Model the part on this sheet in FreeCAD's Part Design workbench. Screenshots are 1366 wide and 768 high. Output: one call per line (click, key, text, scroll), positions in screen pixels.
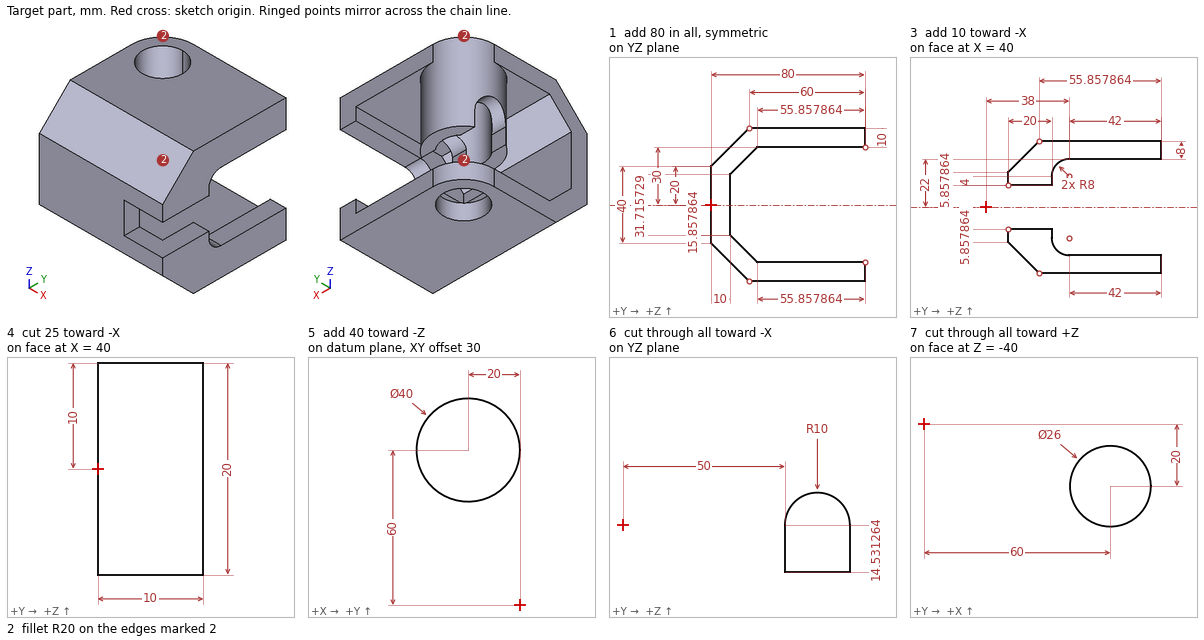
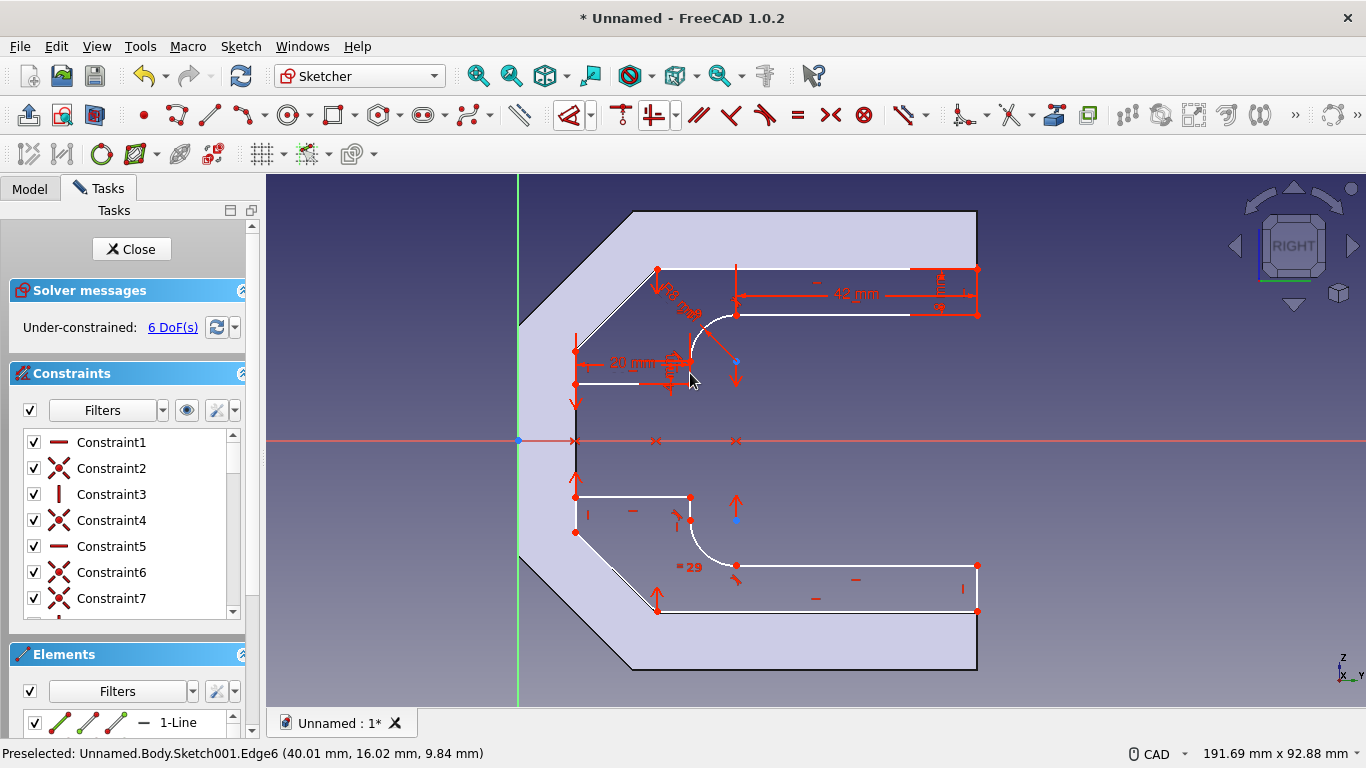
click(905, 566)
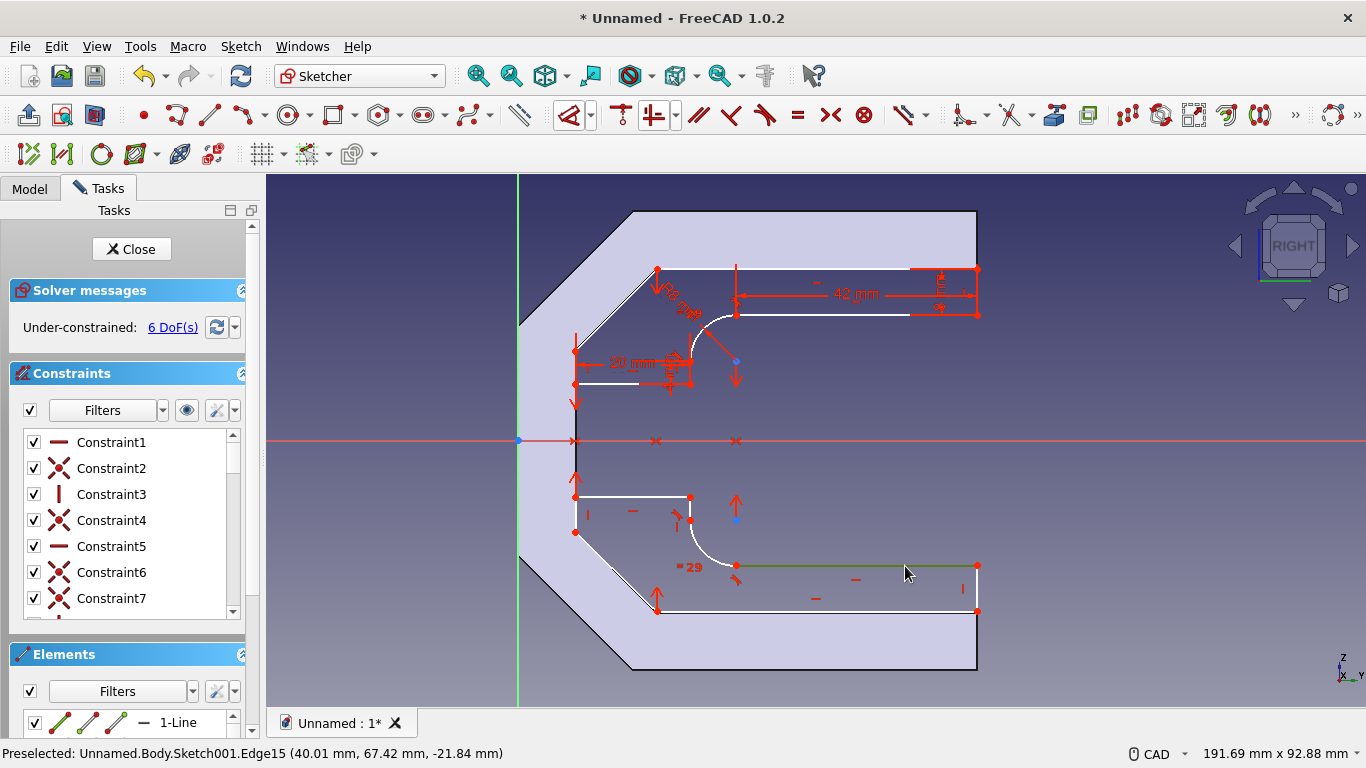
key(l)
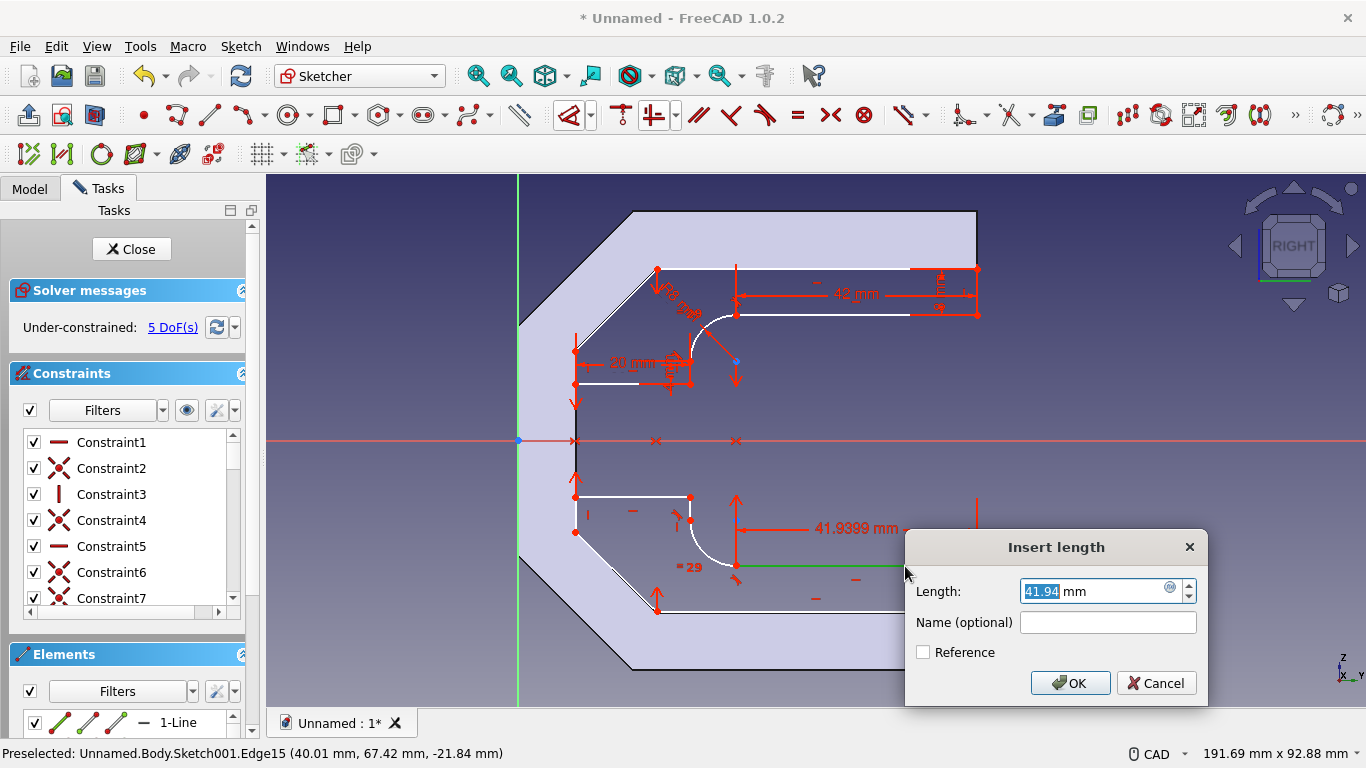
text(42)
key(Return)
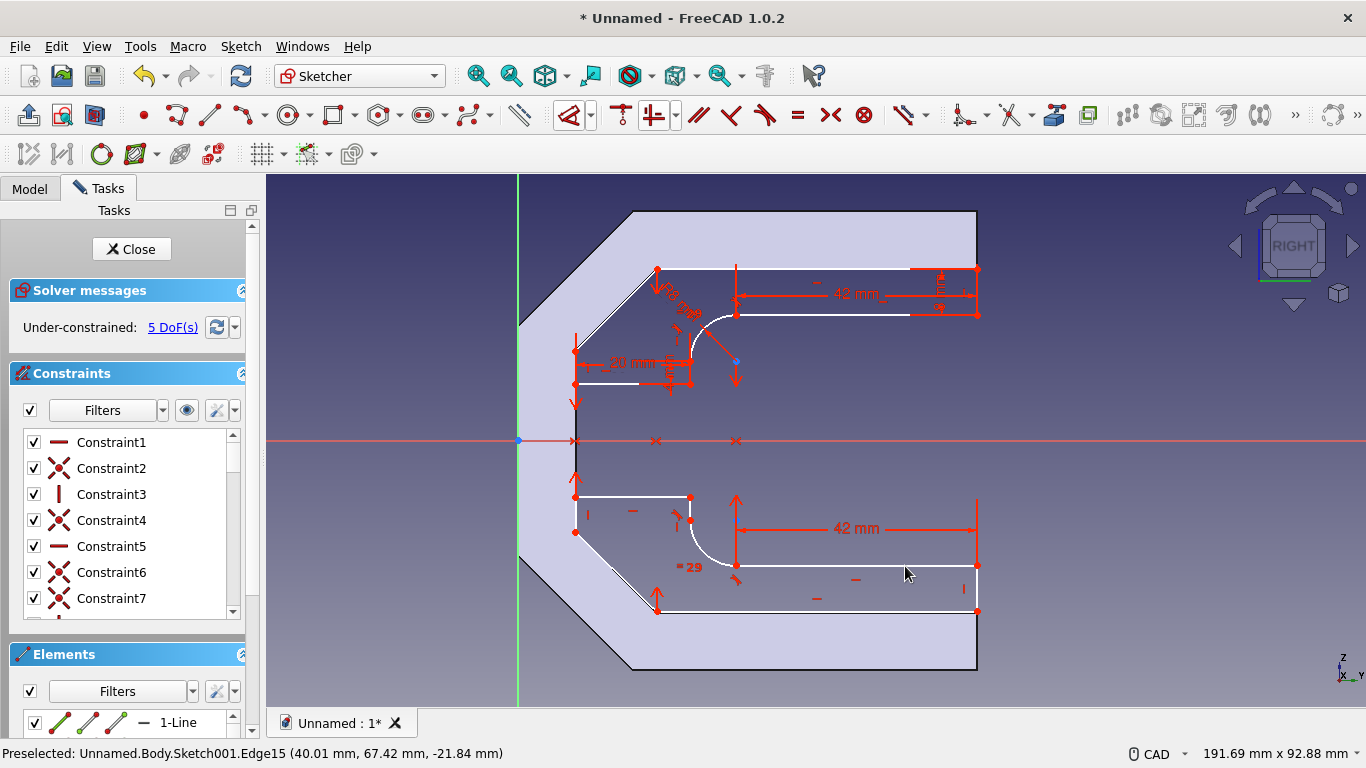
click(736, 315)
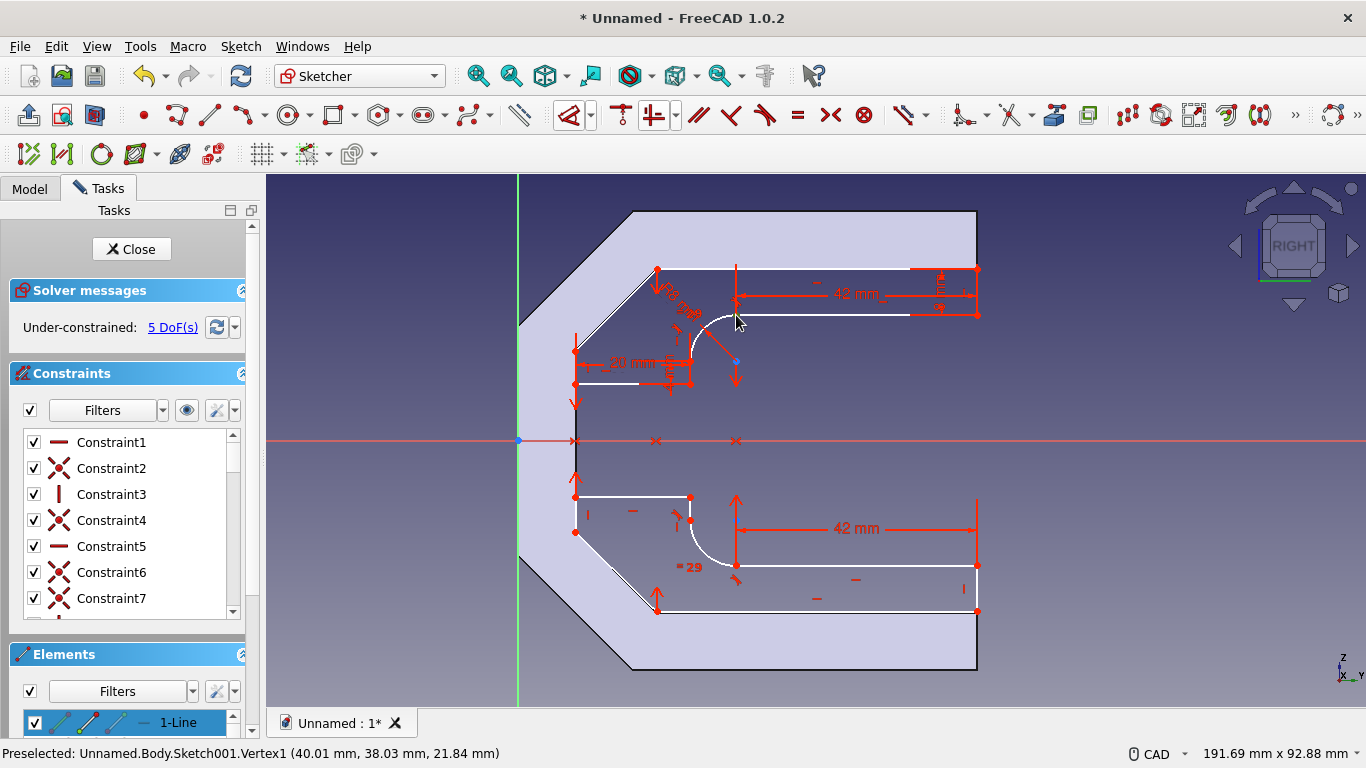
click(590, 116)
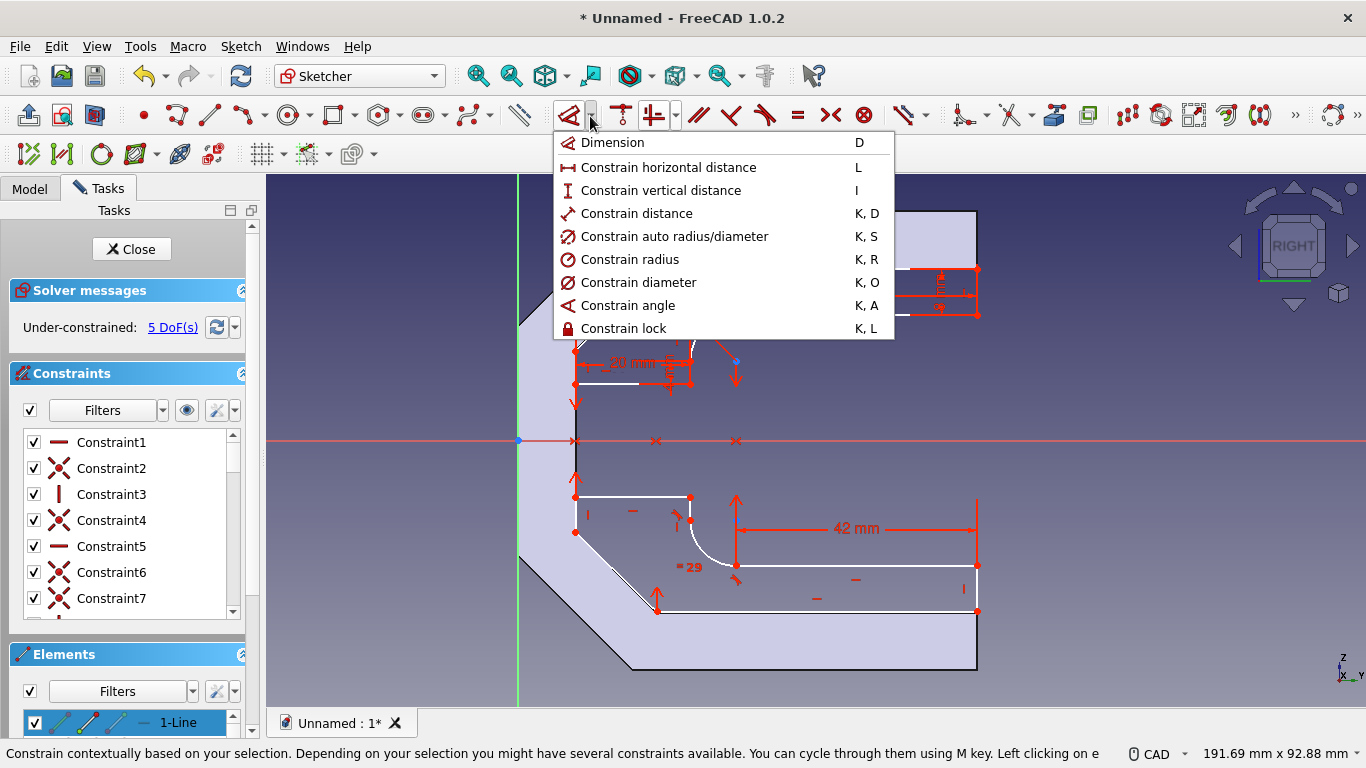
click(724, 168)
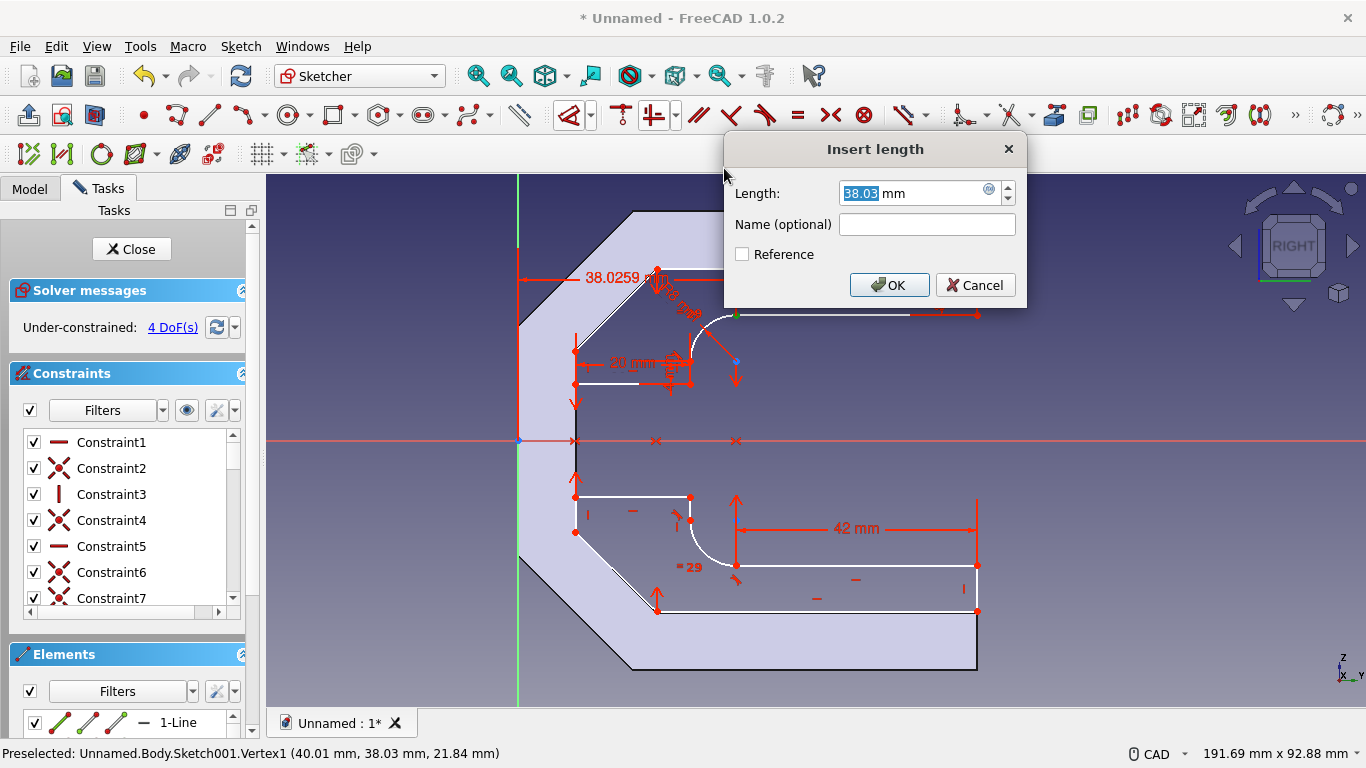
text(38)
key(Return)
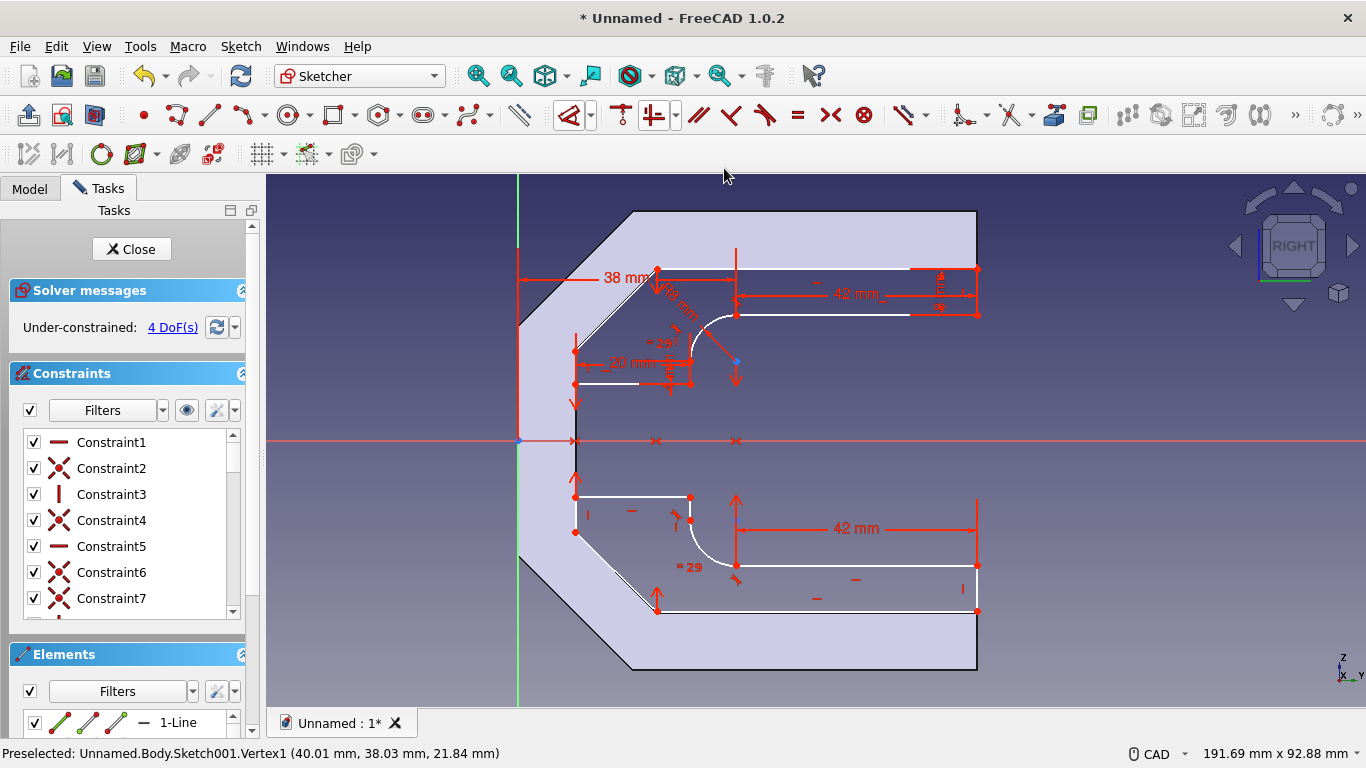
click(736, 315)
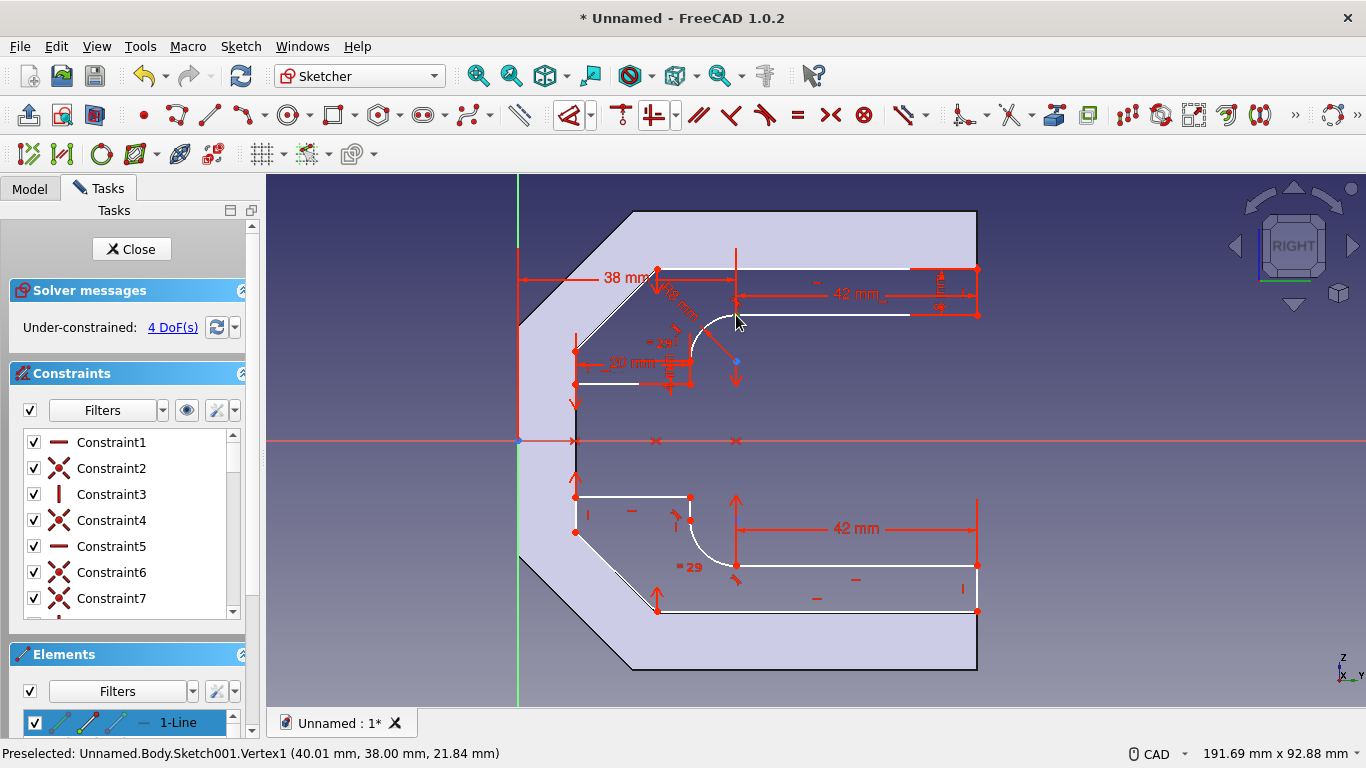
key(i)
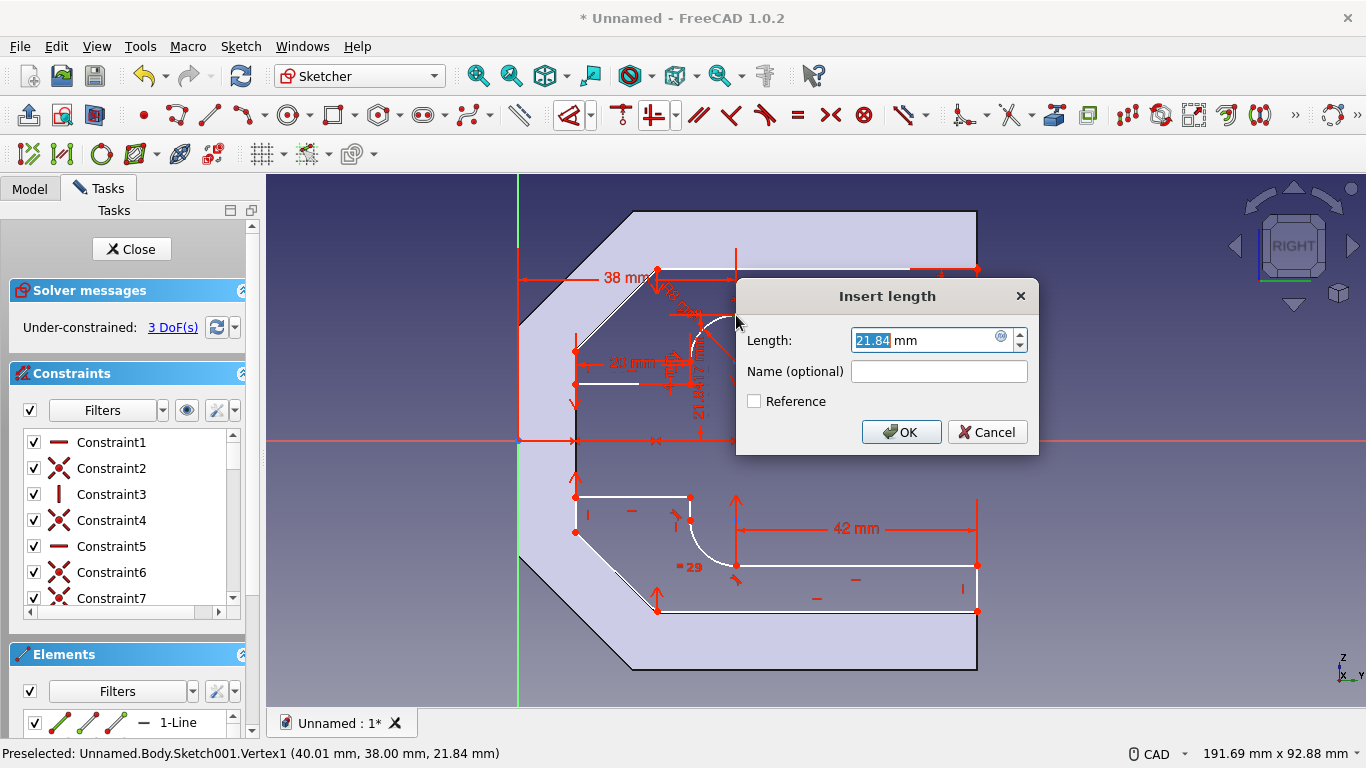
text(22)
key(Return)